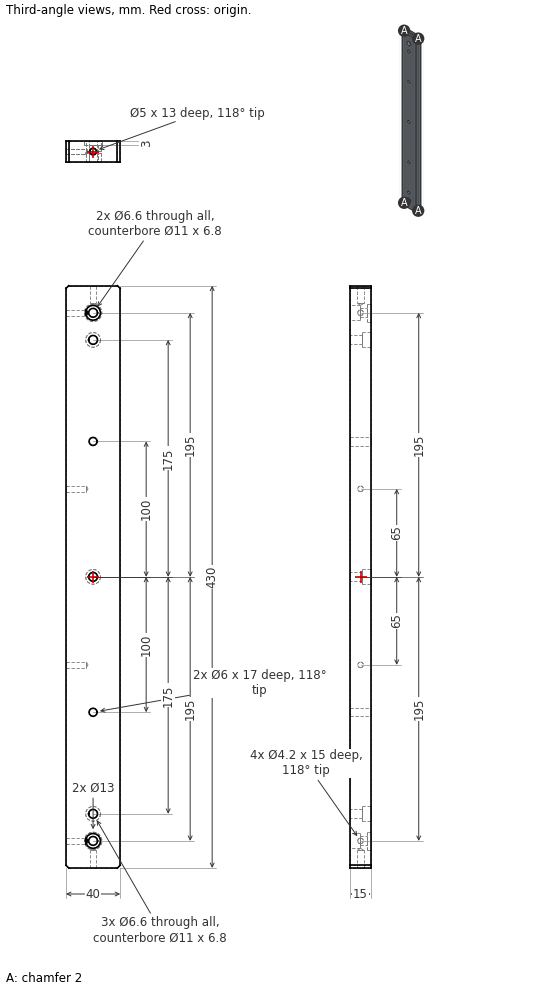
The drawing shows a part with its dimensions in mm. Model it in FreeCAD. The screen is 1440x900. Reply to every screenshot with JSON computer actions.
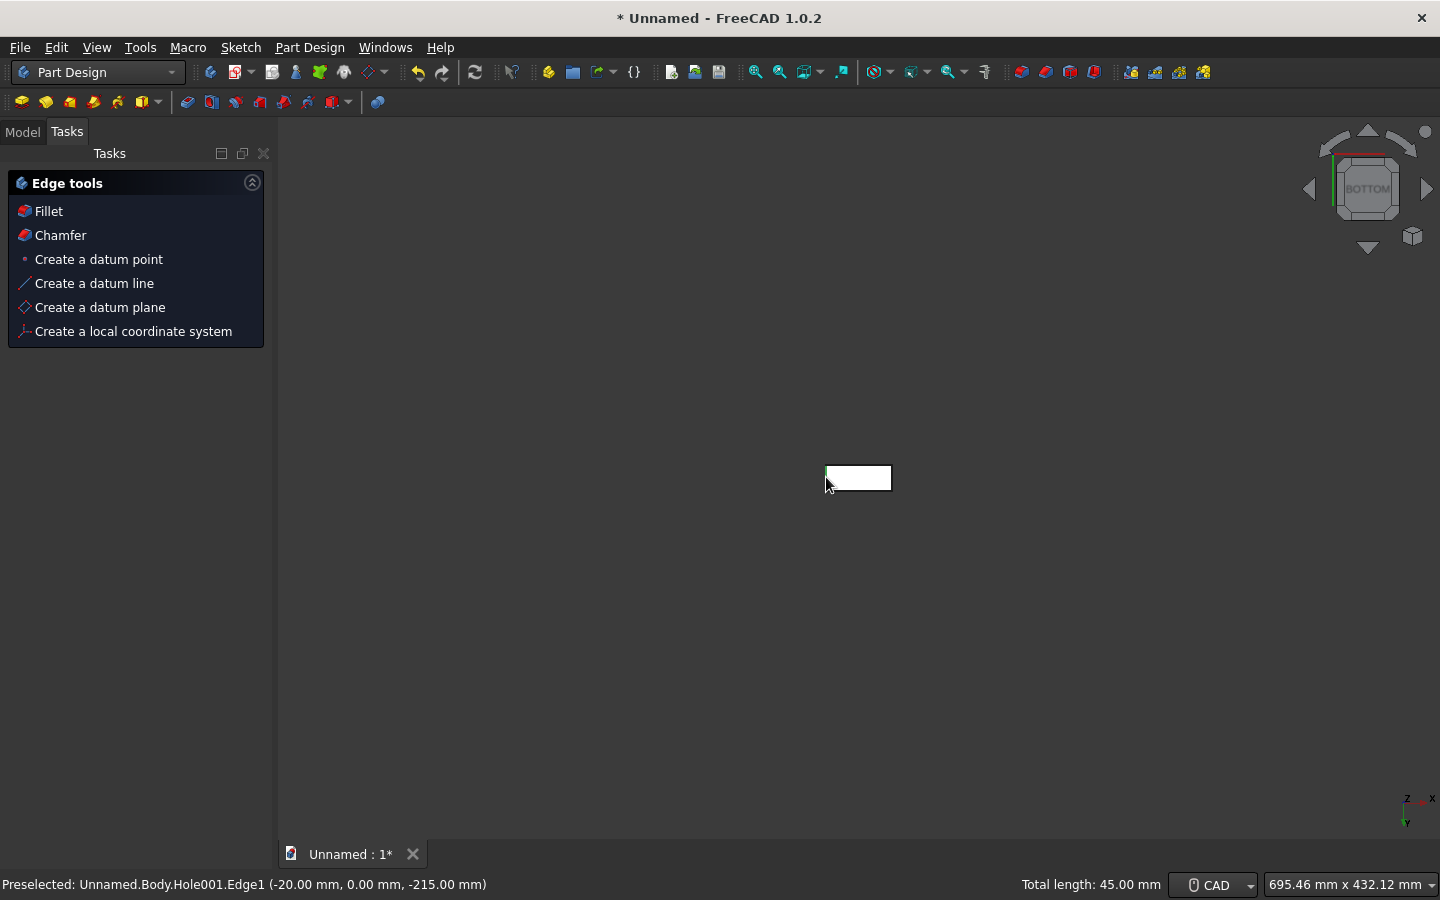
{"action": "left_click", "coordinate": [892, 477], "text": "ctrl"}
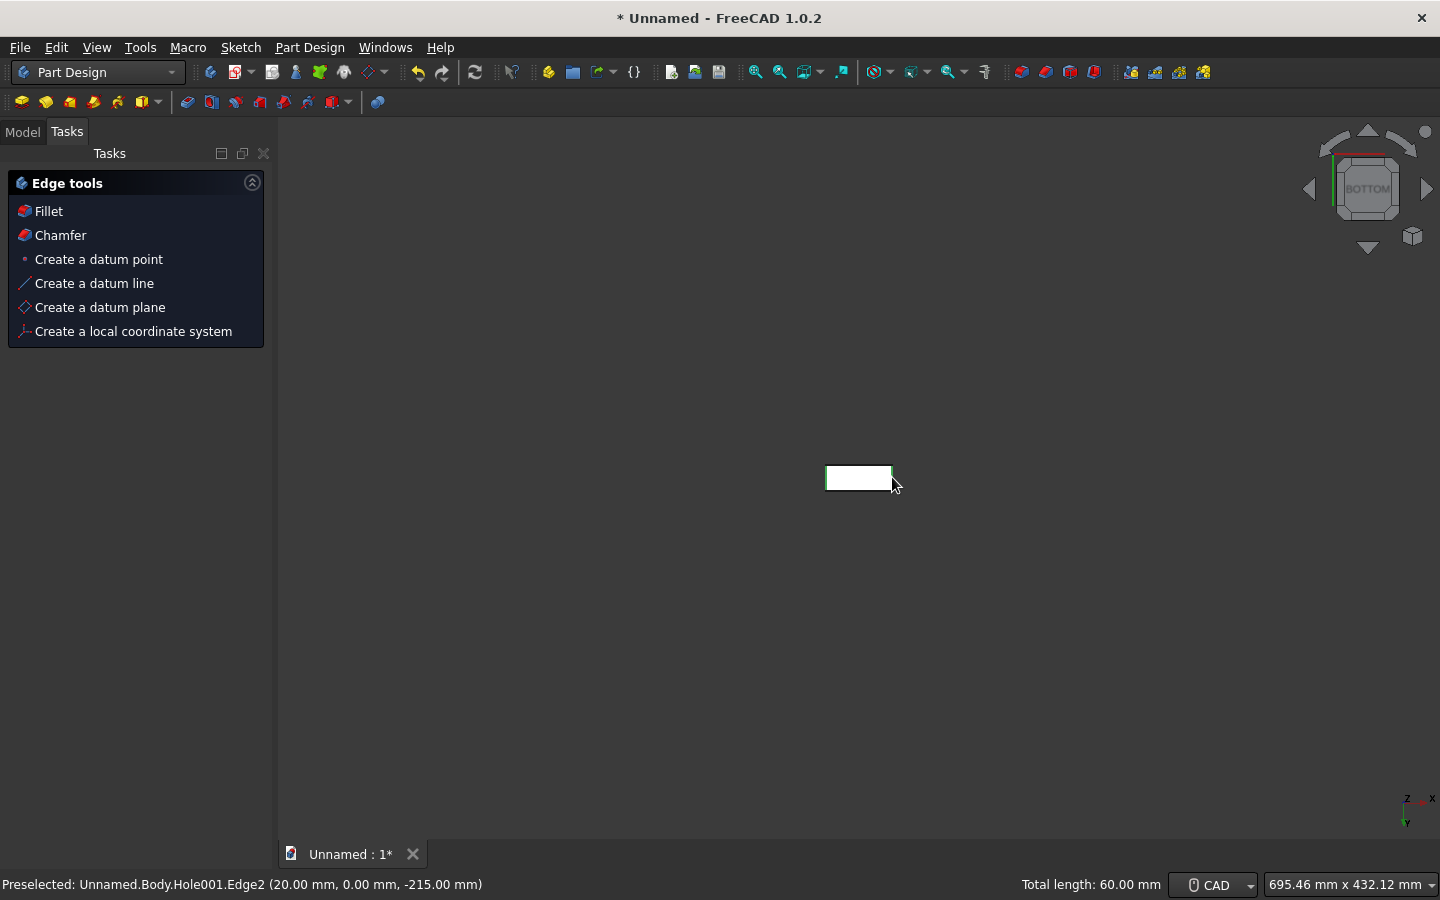
{"action": "left_click", "coordinate": [1046, 72]}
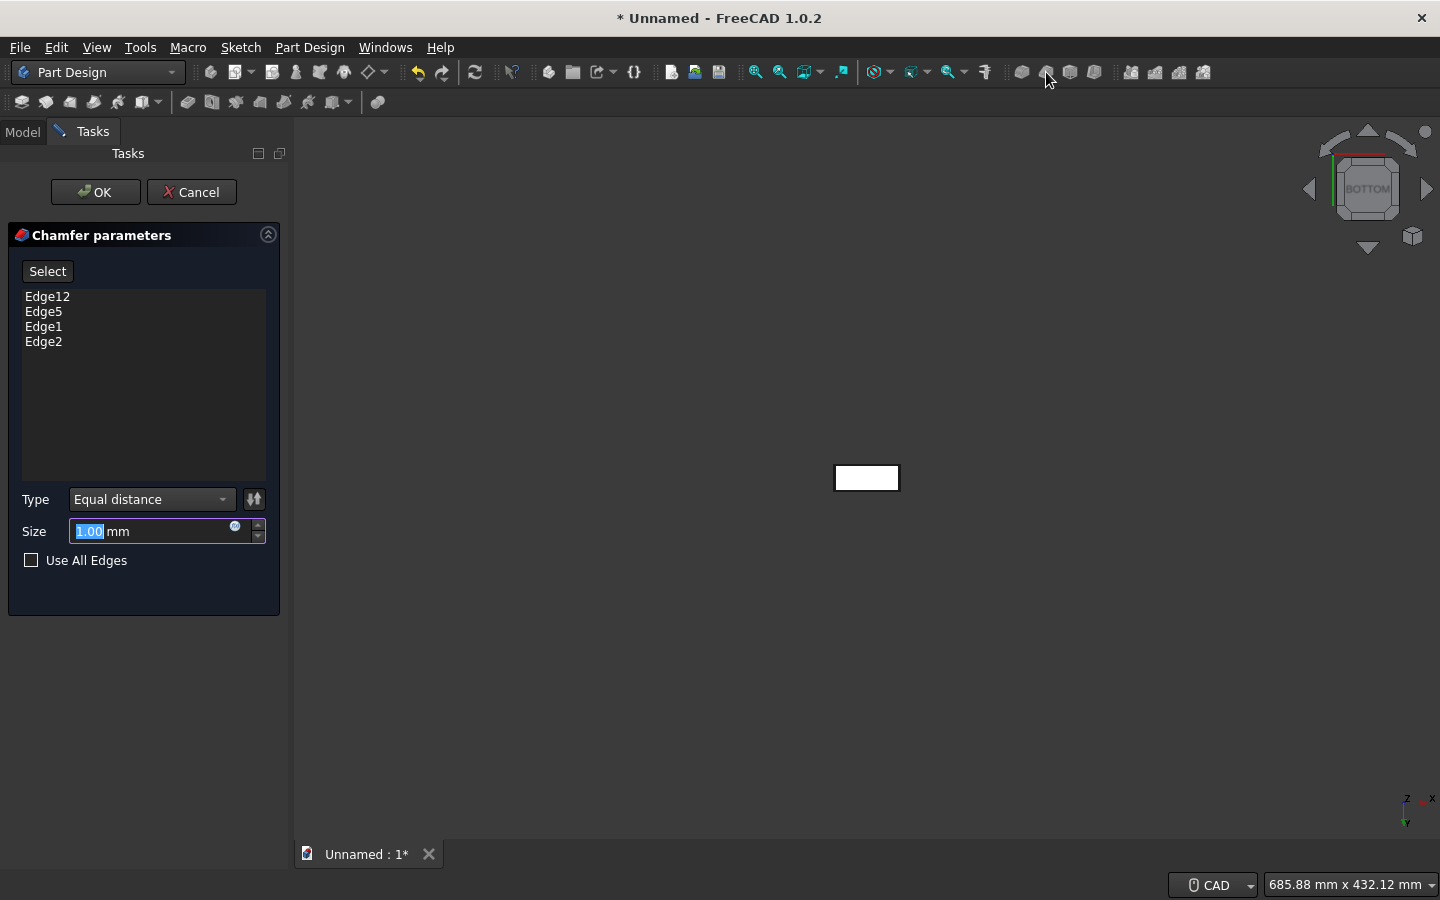
{"action": "type", "text": "2"}
{"action": "key", "text": "Tab"}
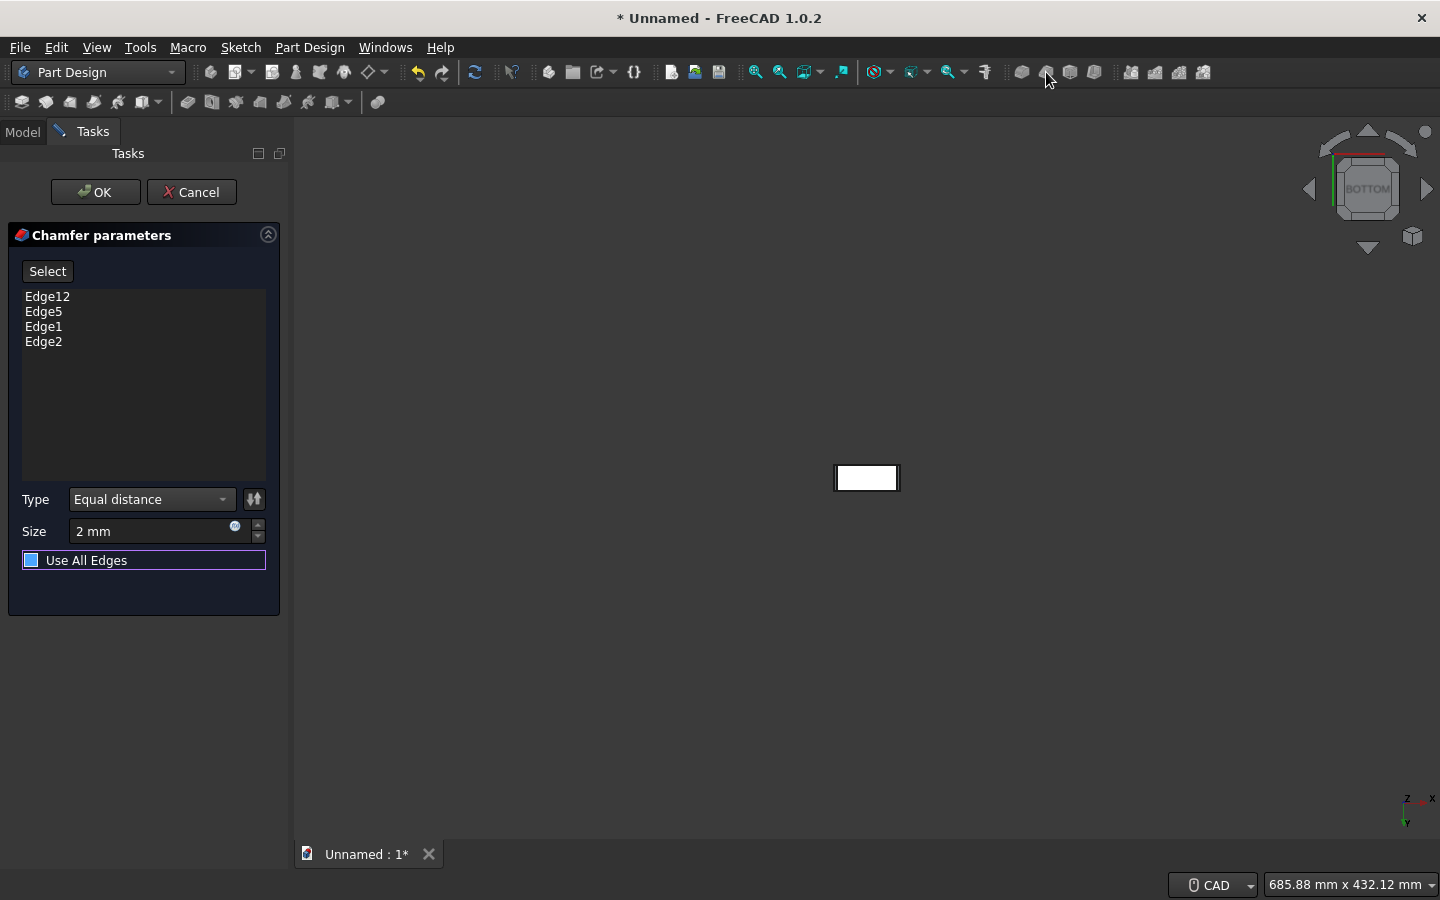
{"action": "left_click", "coordinate": [96, 192]}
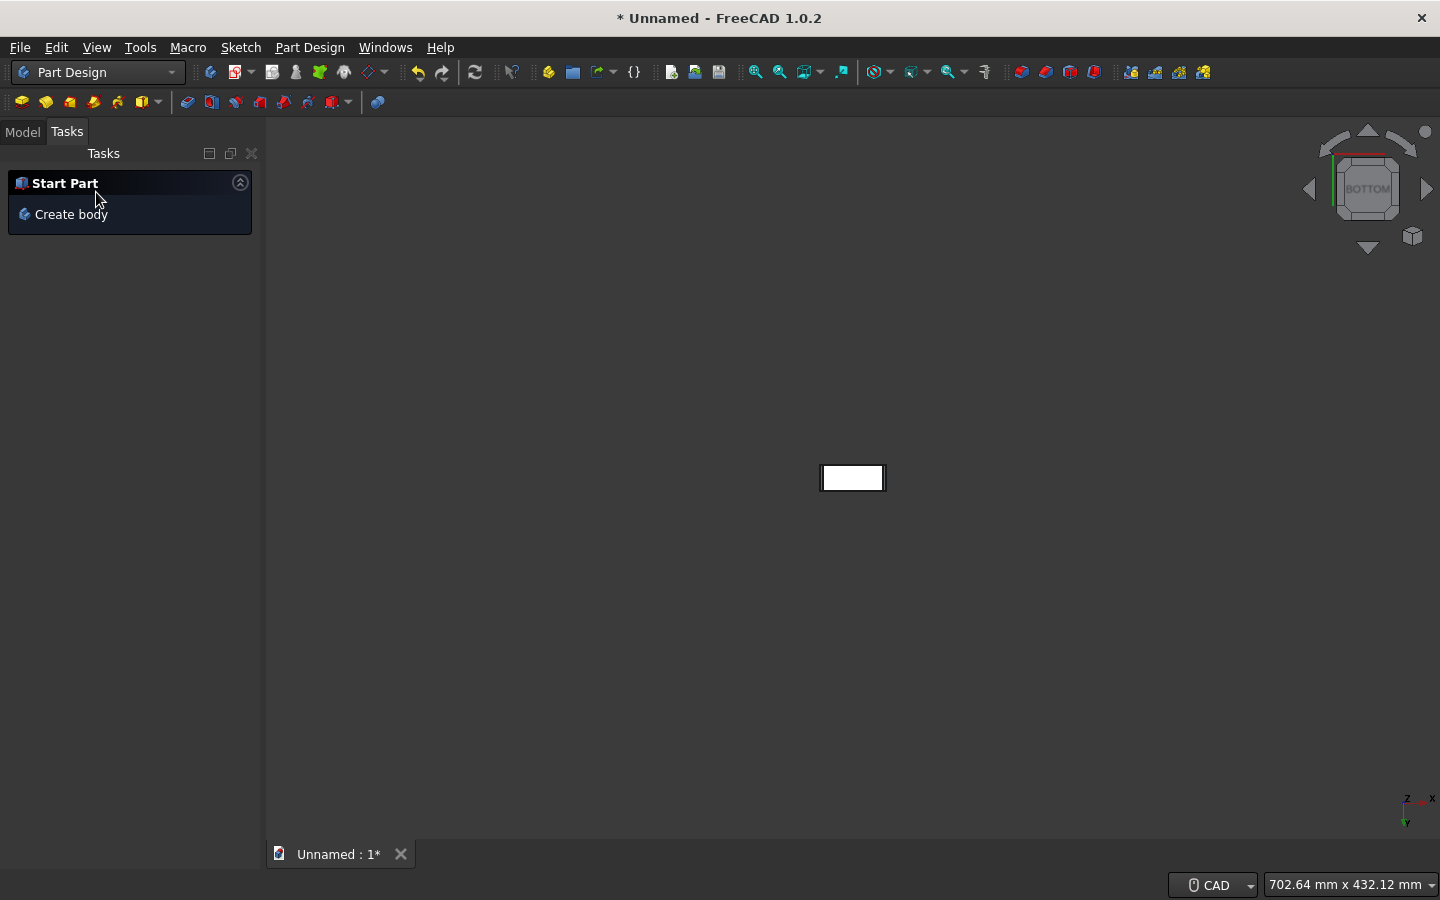
{"action": "left_click", "coordinate": [756, 72]}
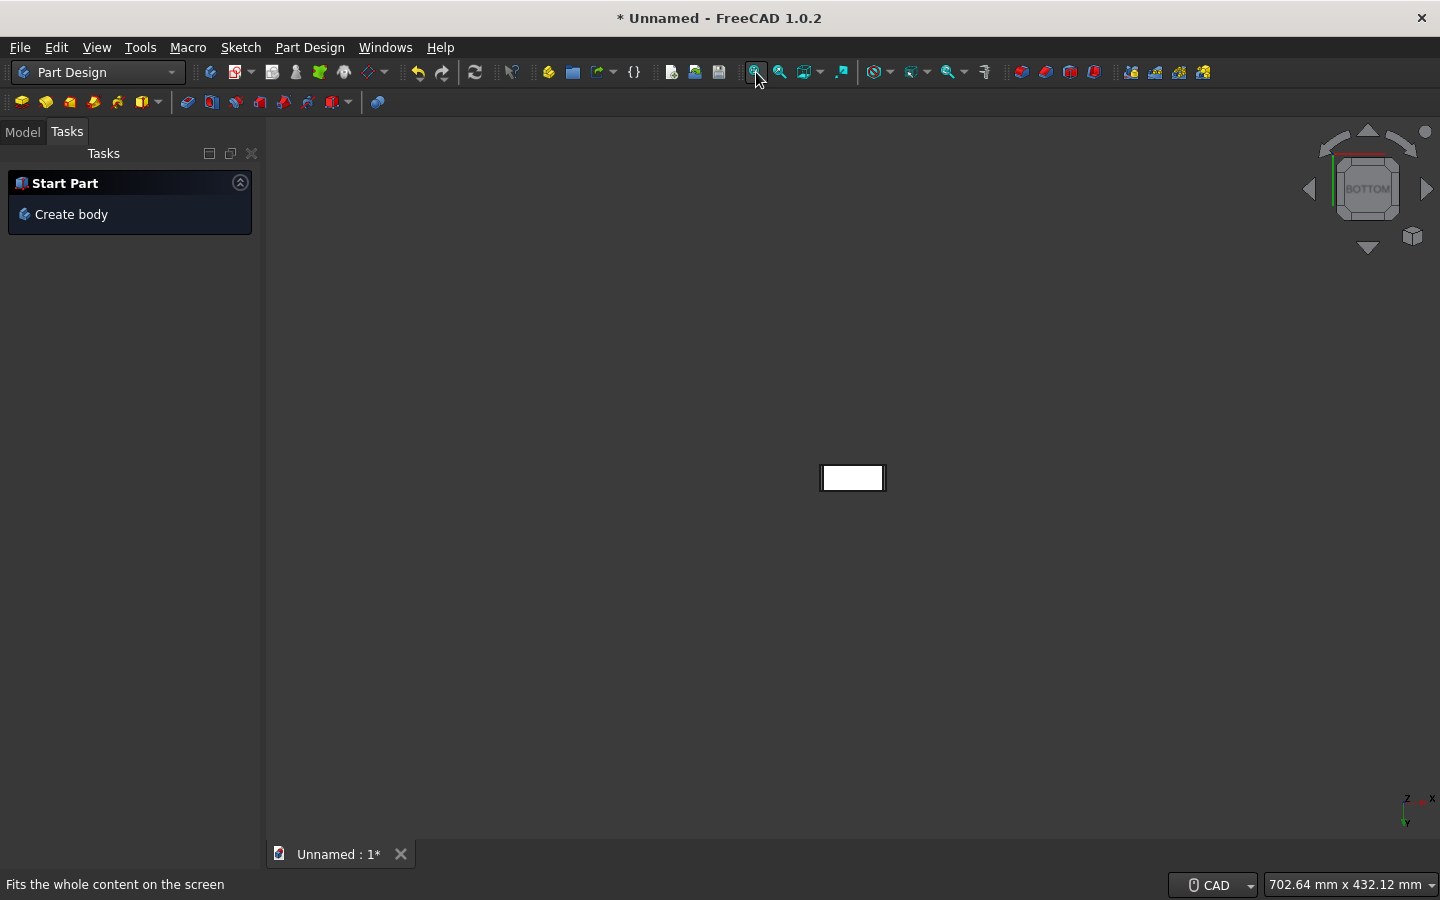
{"action": "key", "text": "4"}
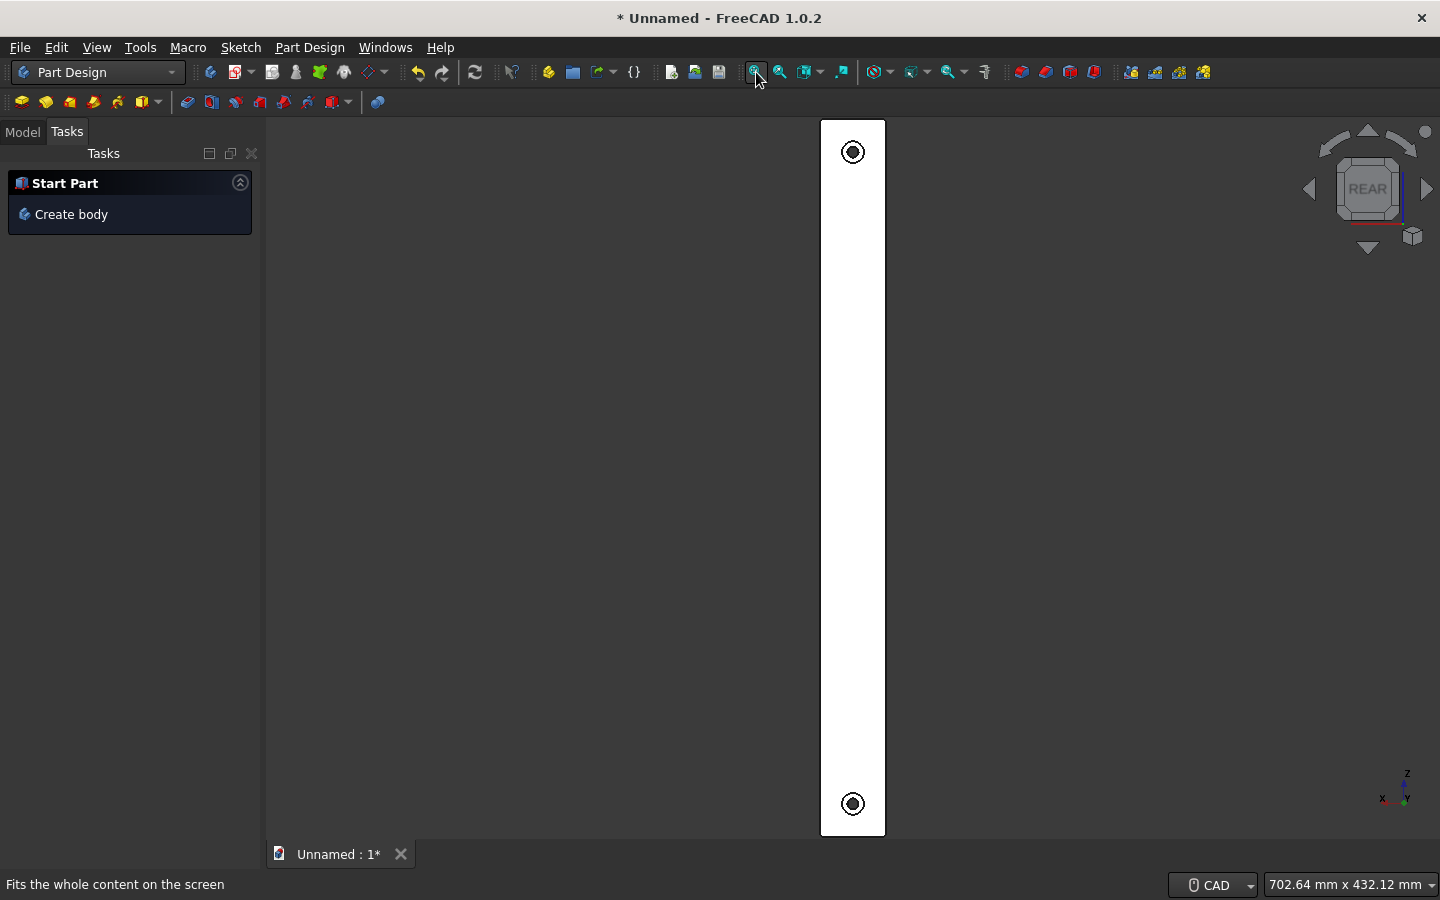
{"action": "left_click", "coordinate": [853, 272]}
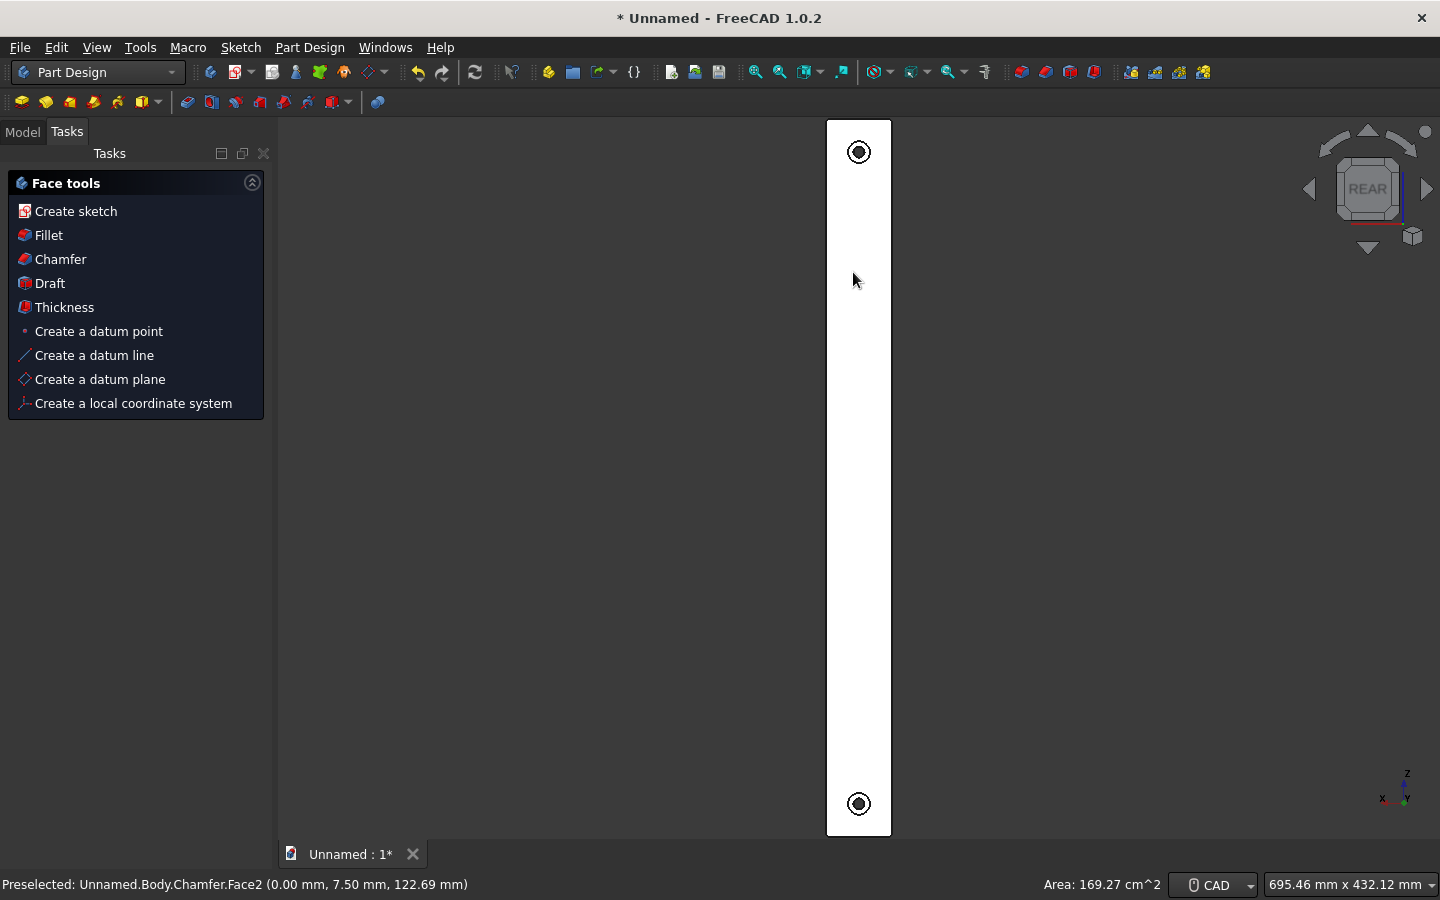
{"action": "left_click", "coordinate": [236, 72]}